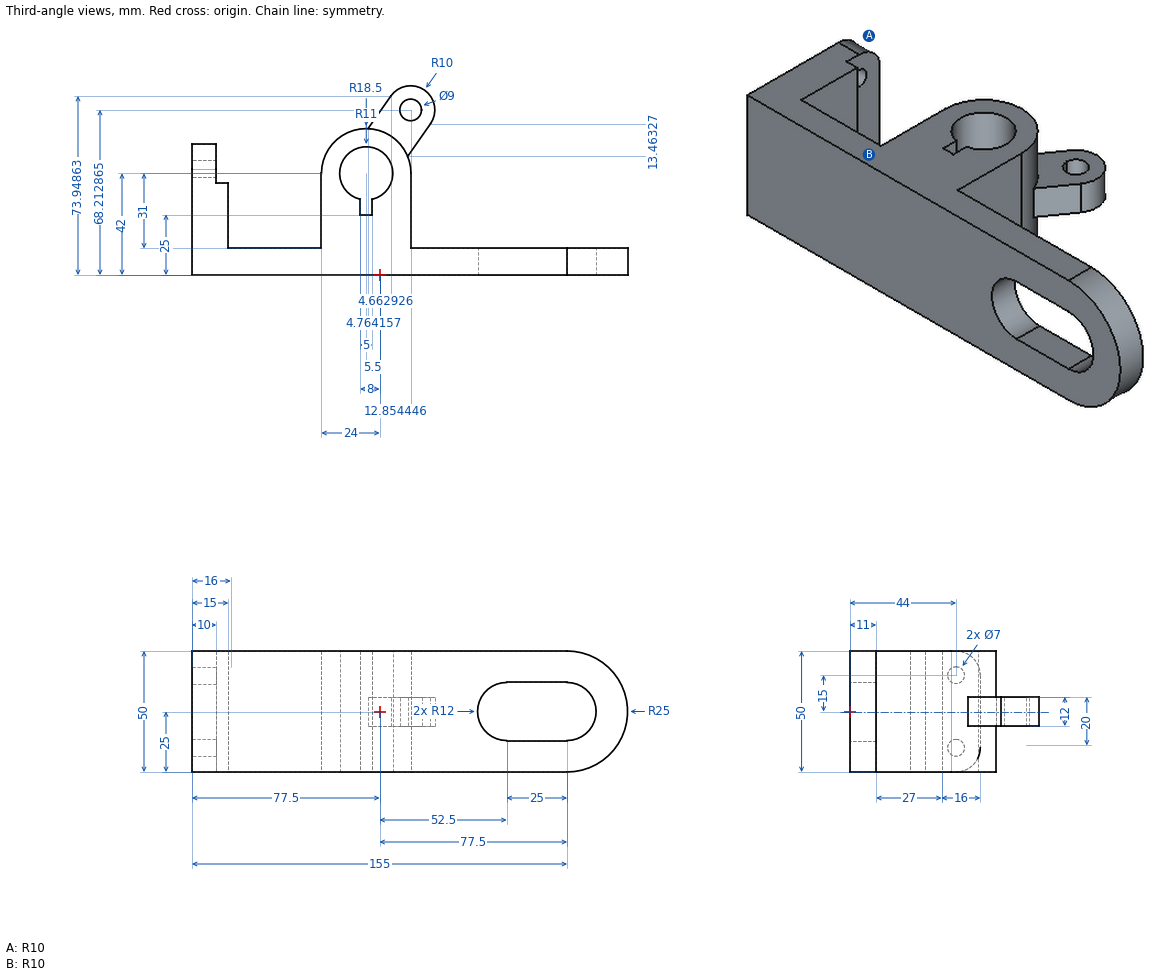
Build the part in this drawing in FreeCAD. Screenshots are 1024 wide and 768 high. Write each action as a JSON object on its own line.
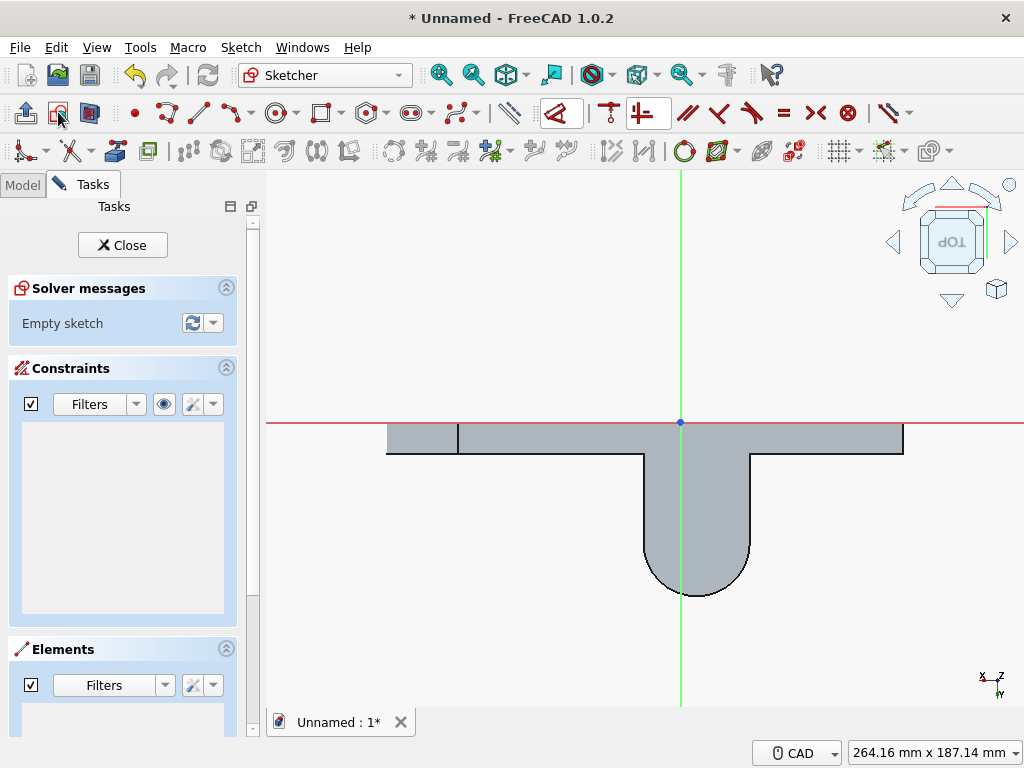
{"action": "scroll", "coordinate": [787, 548], "scroll_direction": "up", "scroll_amount": 4}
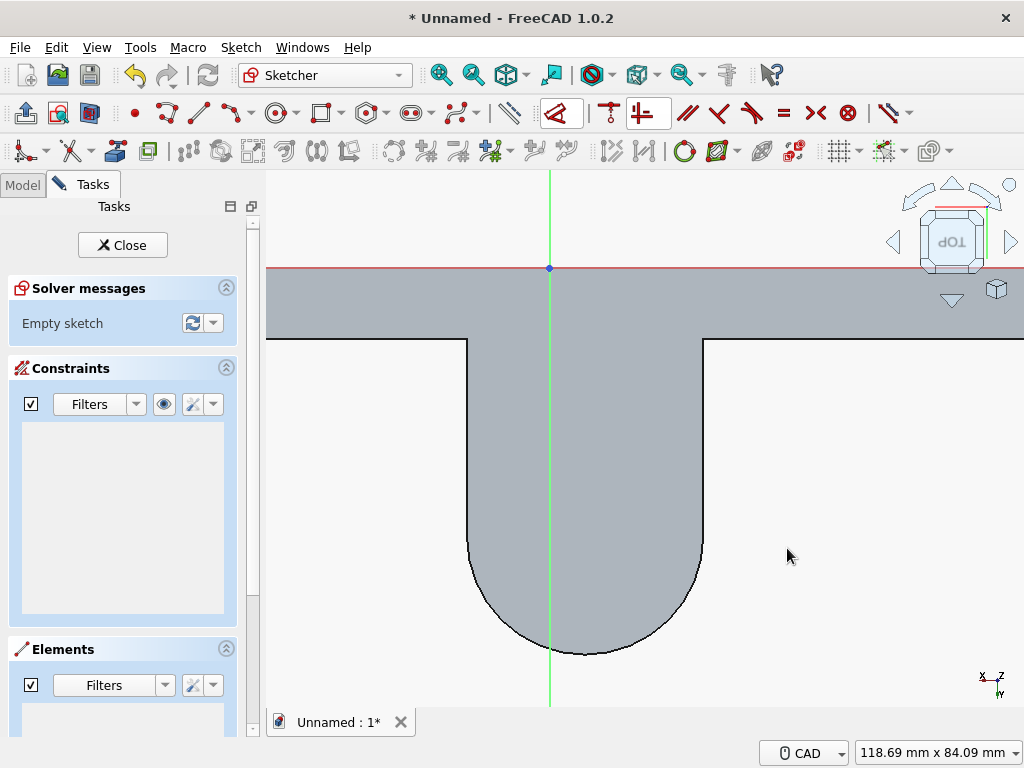
{"action": "left_click", "coordinate": [168, 114]}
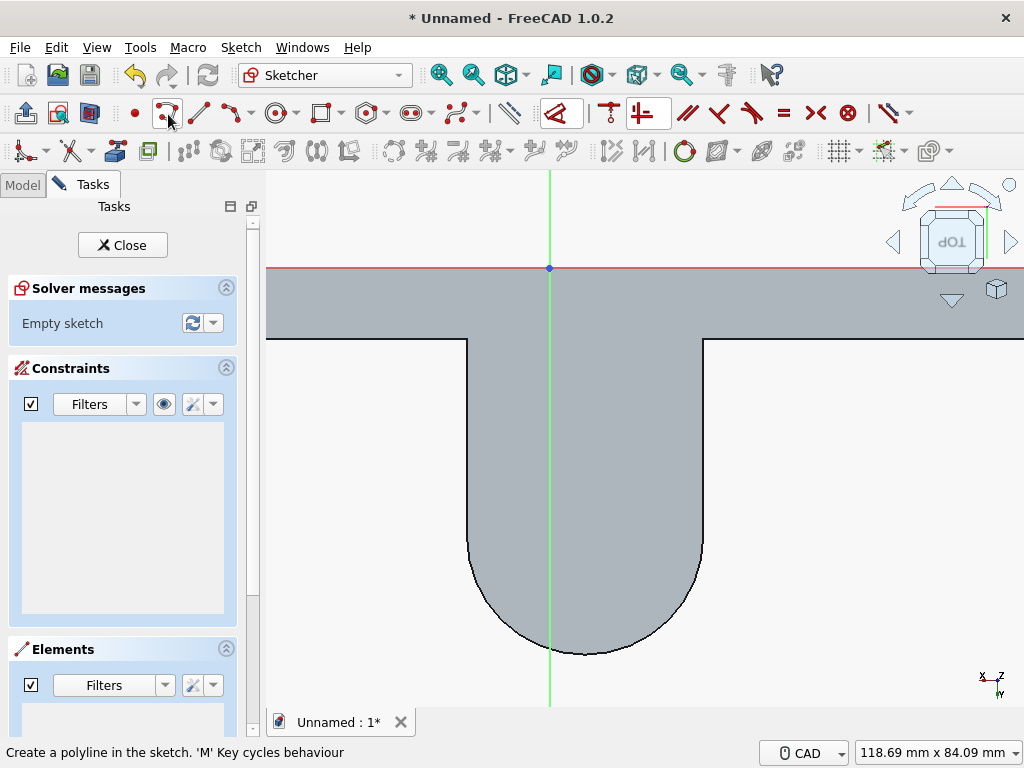
{"action": "left_click", "coordinate": [601, 468]}
{"action": "left_click", "coordinate": [601, 428]}
{"action": "left_click", "coordinate": [569, 428]}
{"action": "left_click", "coordinate": [569, 468]}
{"action": "right_click", "coordinate": [569, 468]}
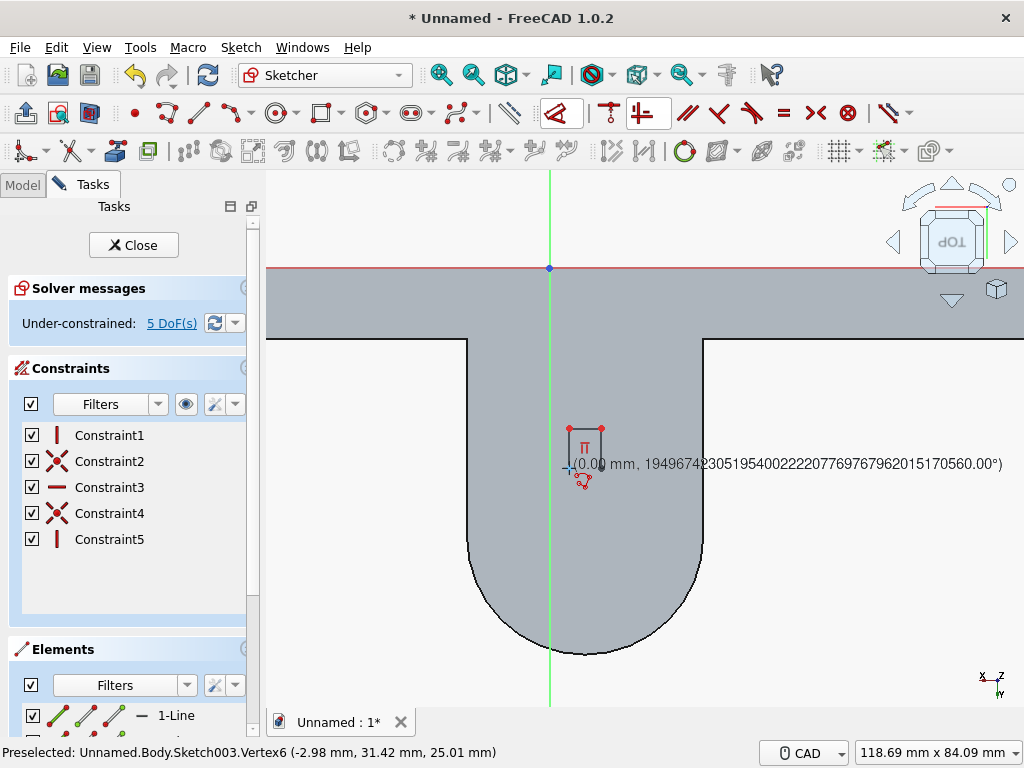
{"action": "left_click", "coordinate": [232, 114]}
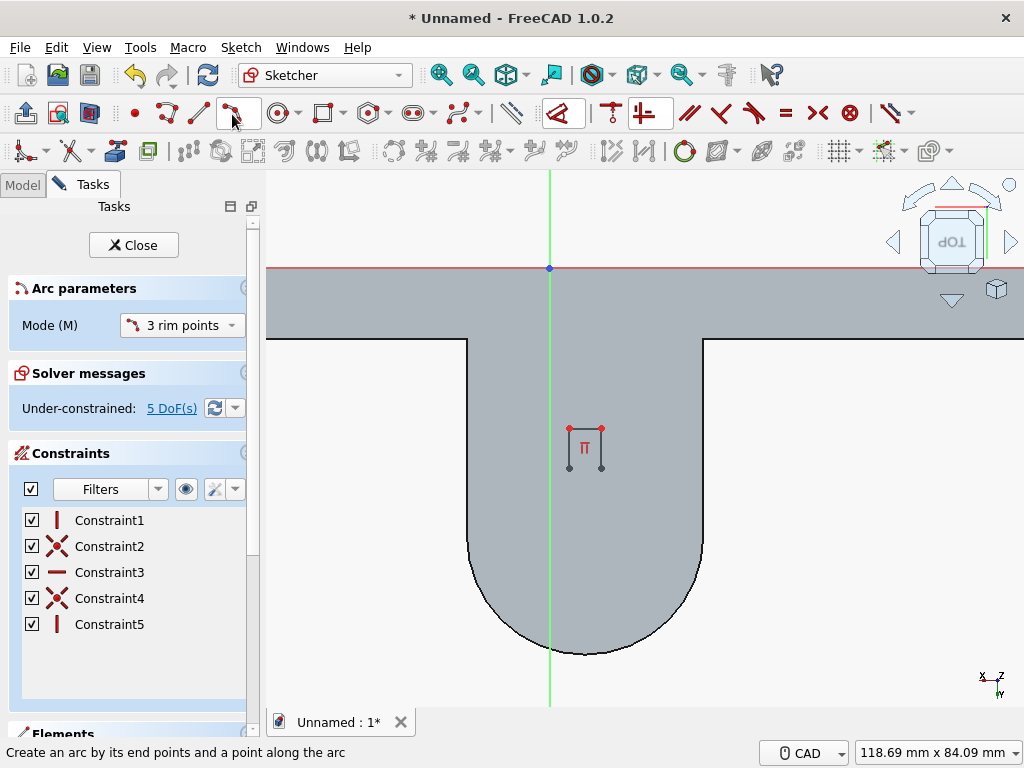
{"action": "left_click", "coordinate": [569, 469]}
{"action": "left_click", "coordinate": [601, 469]}
{"action": "left_click", "coordinate": [585, 607]}
{"action": "key", "text": "Escape"}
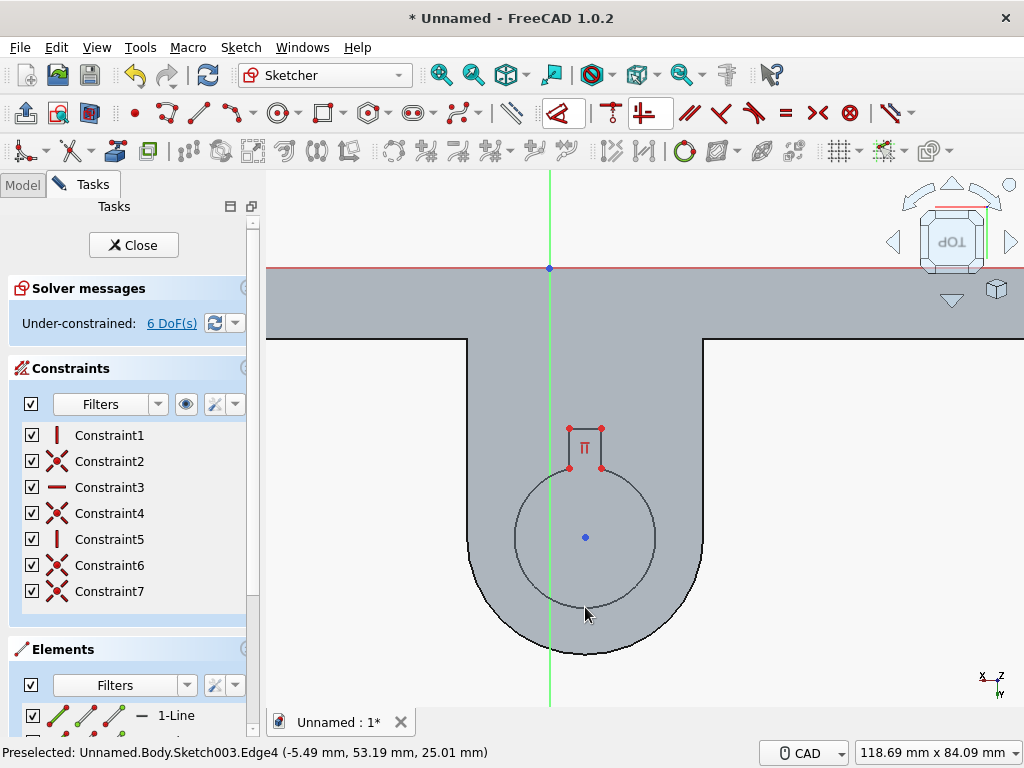
{"action": "left_click", "coordinate": [520, 565]}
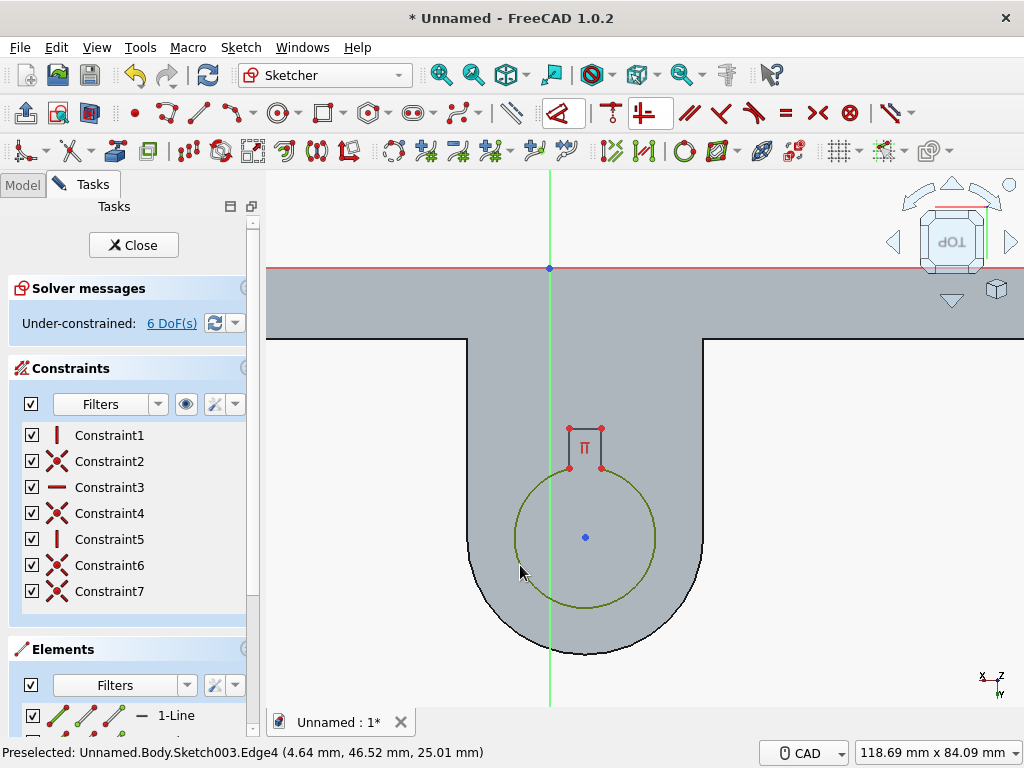
{"action": "left_click", "coordinate": [580, 114]}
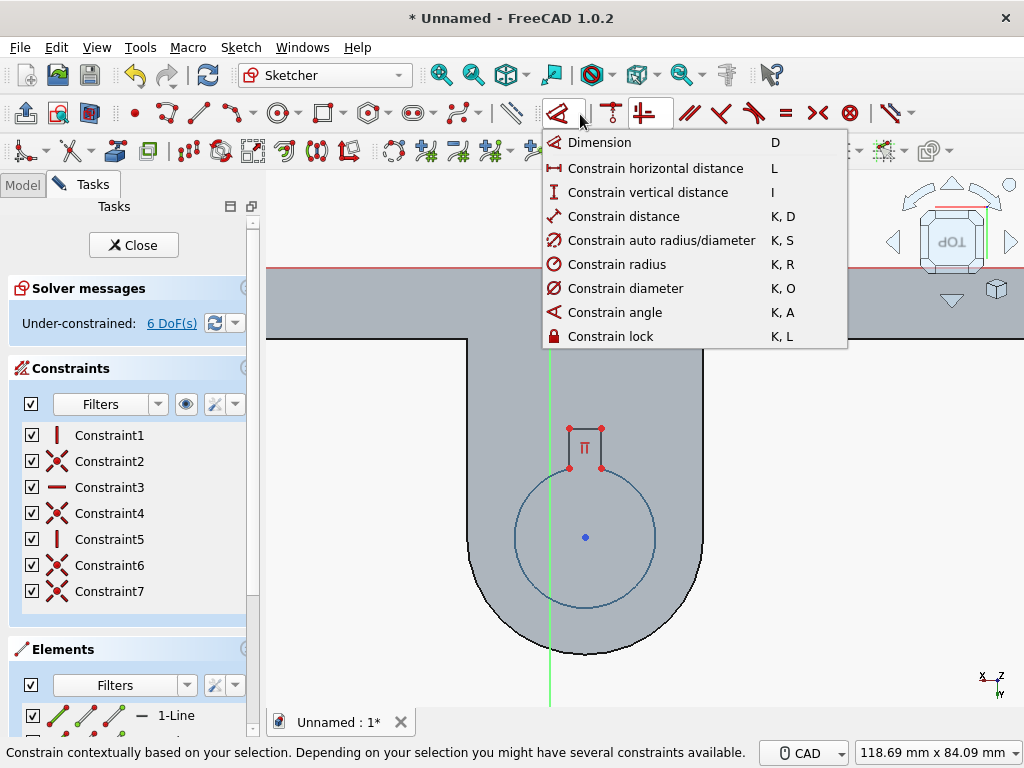
{"action": "left_click", "coordinate": [695, 264]}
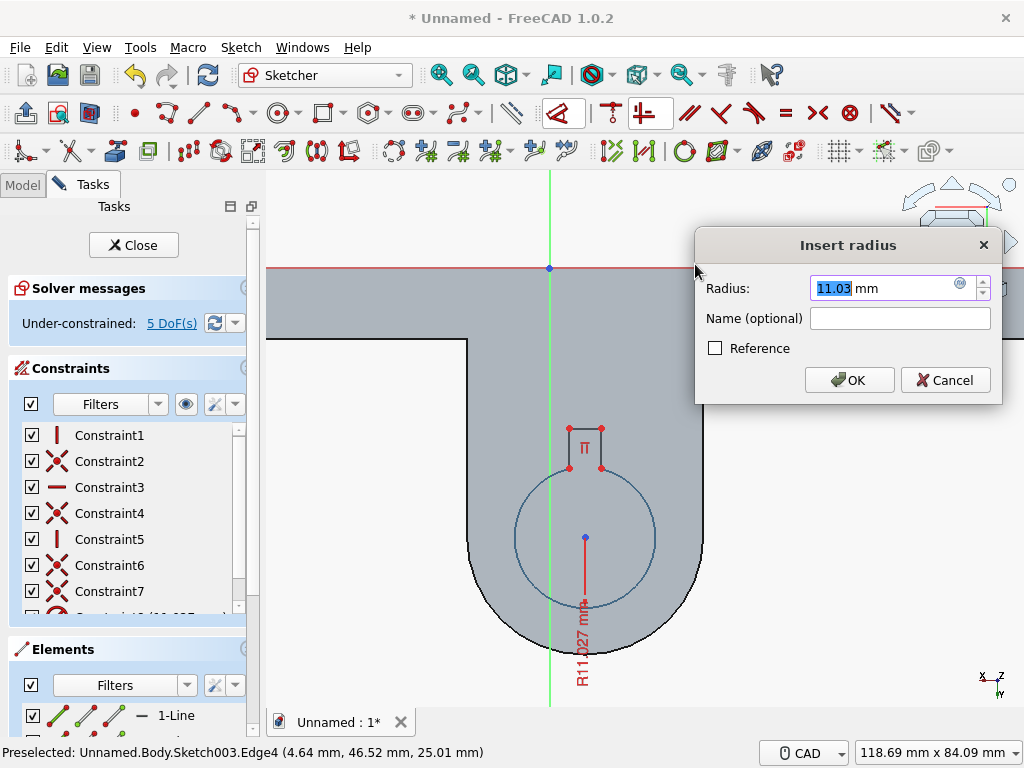
{"action": "type", "text": "11"}
{"action": "key", "text": "Return"}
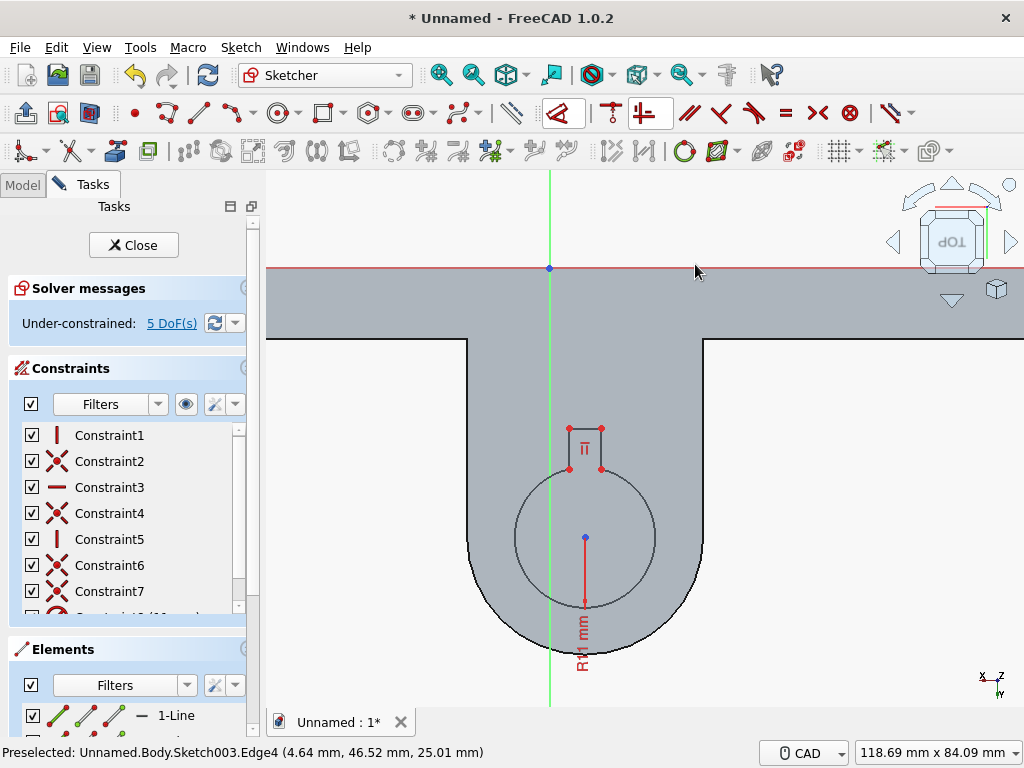
{"action": "scroll", "coordinate": [591, 429], "scroll_direction": "up", "scroll_amount": 2}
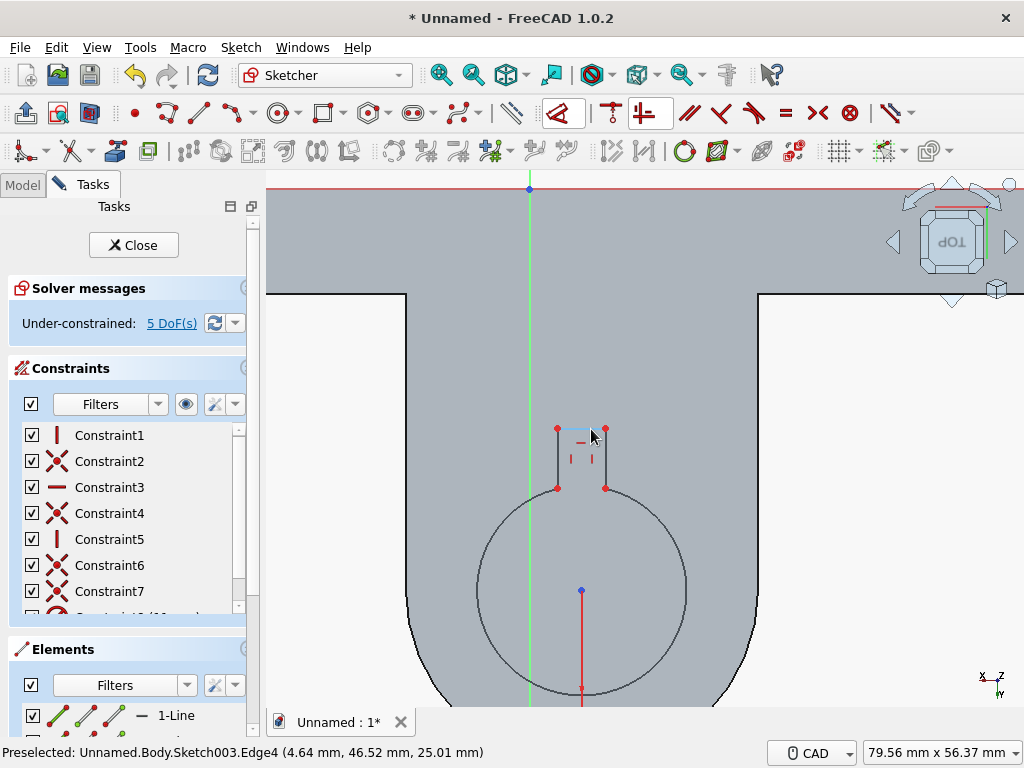
{"action": "left_click", "coordinate": [591, 429]}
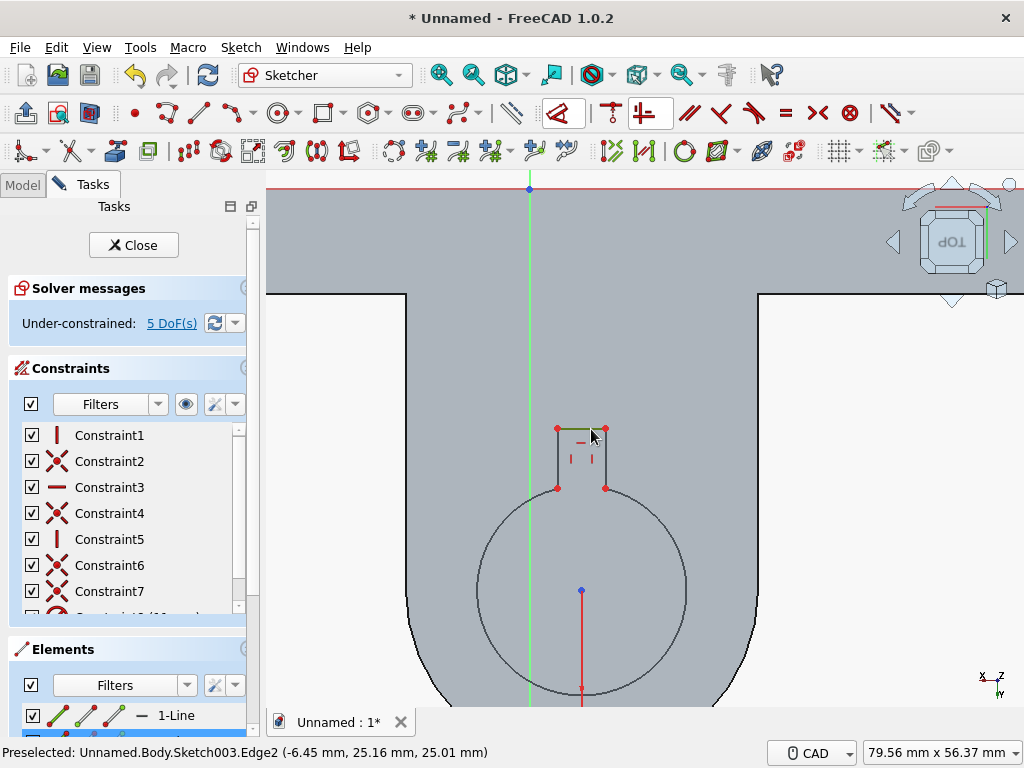
{"action": "key", "text": "l"}